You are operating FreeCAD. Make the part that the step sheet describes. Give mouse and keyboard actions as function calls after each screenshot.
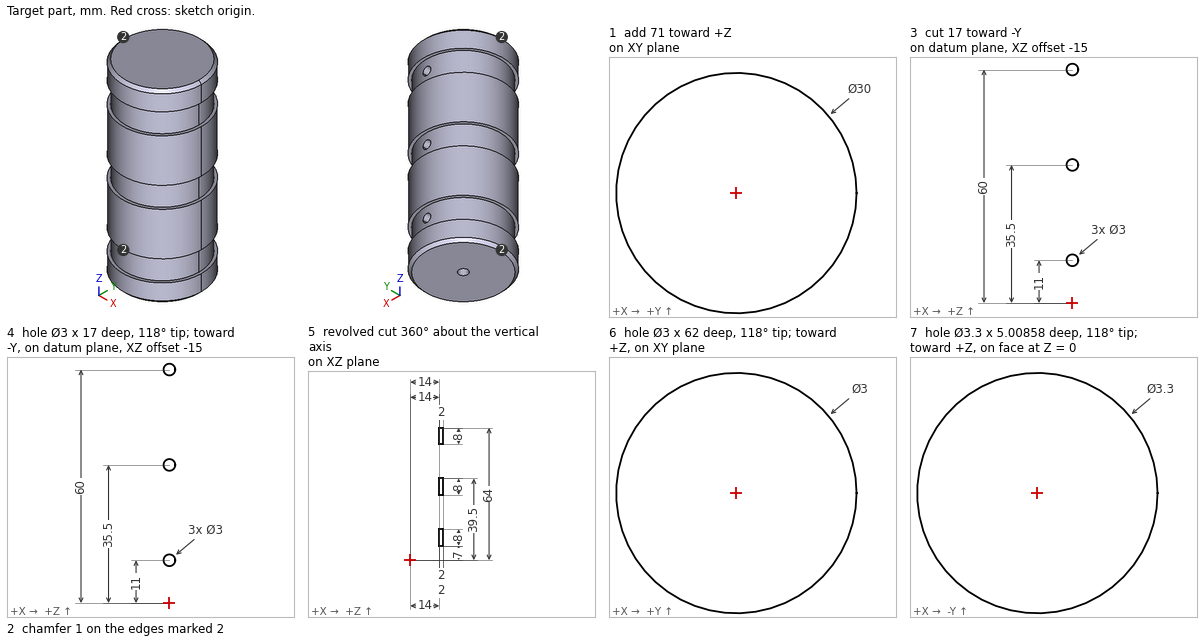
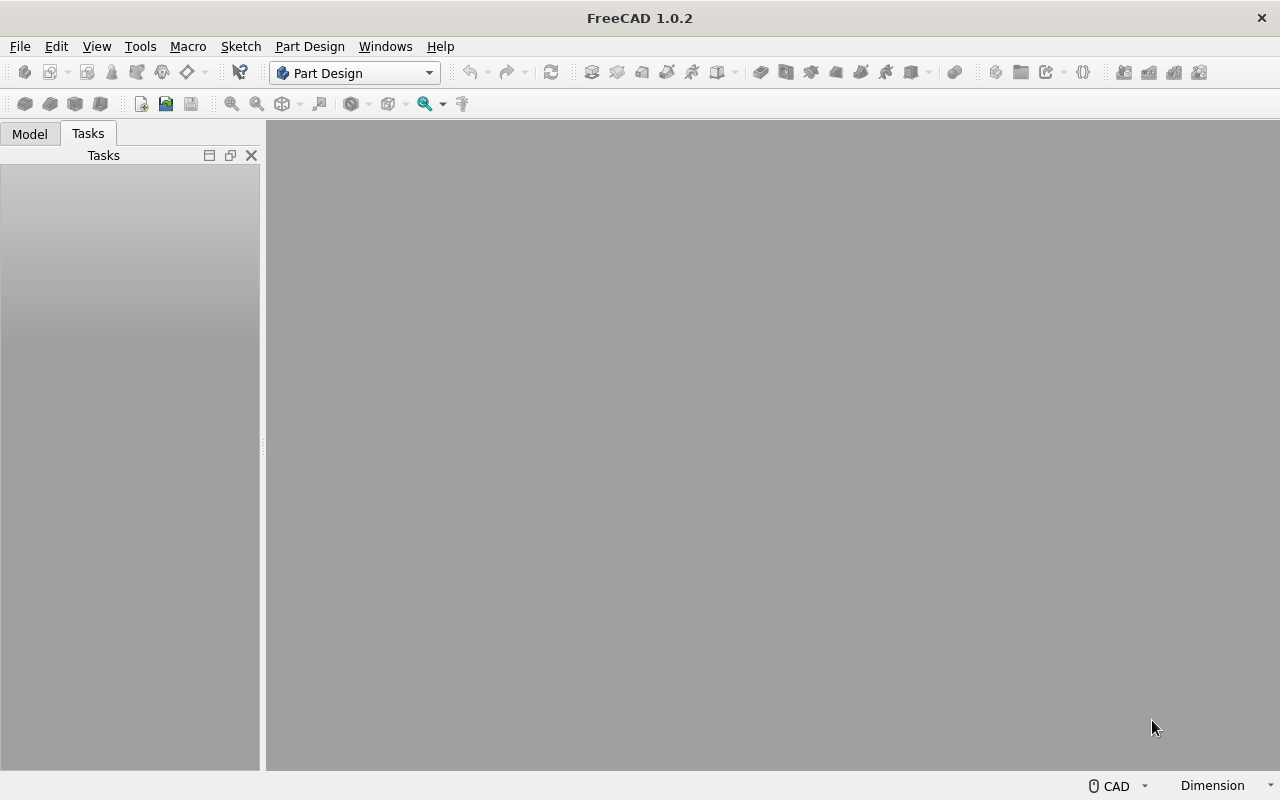
click(141, 104)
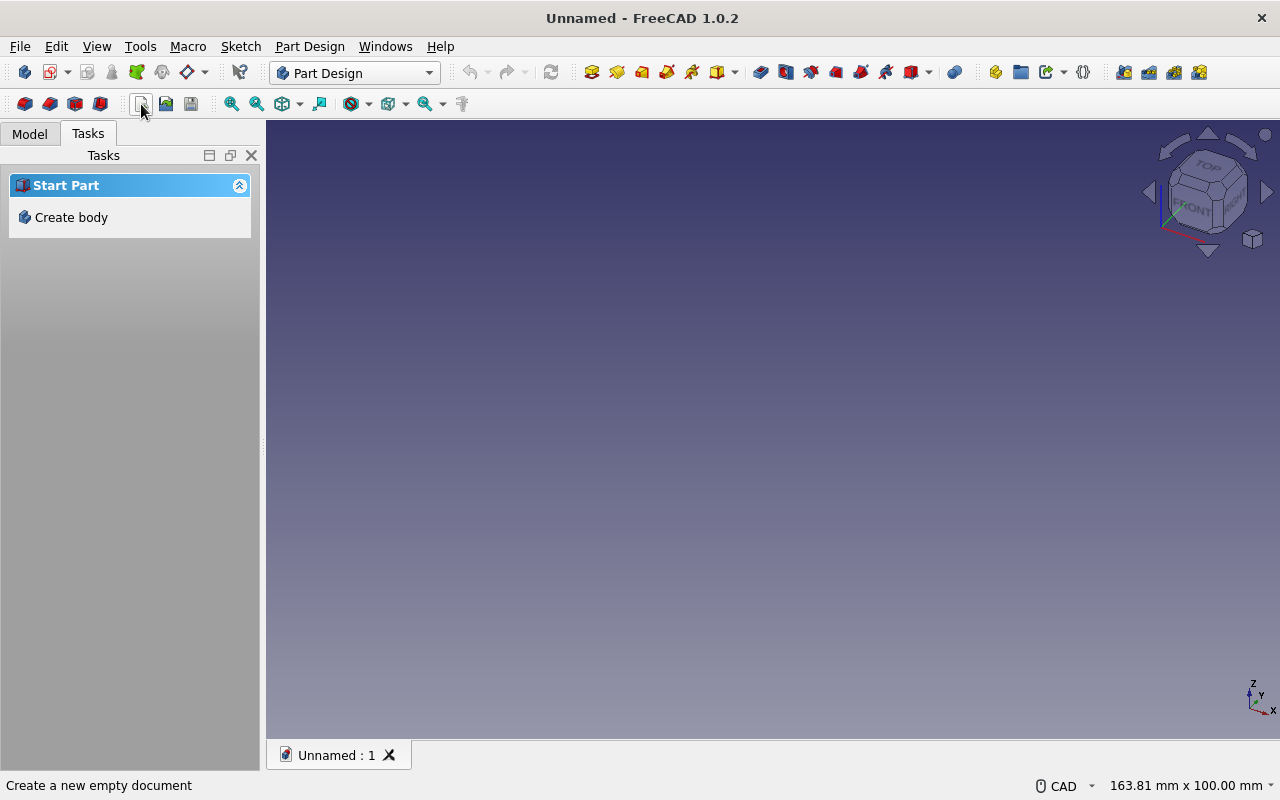
click(50, 72)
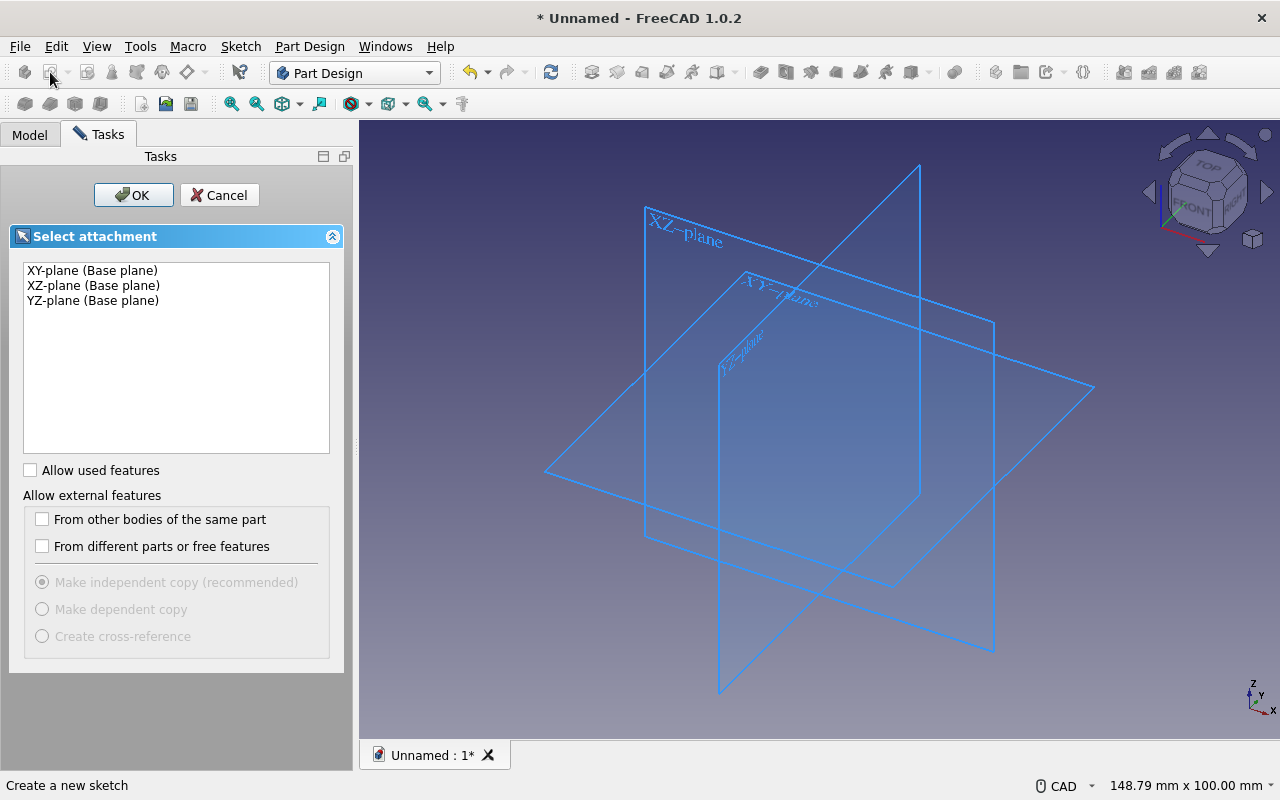
click(84, 270)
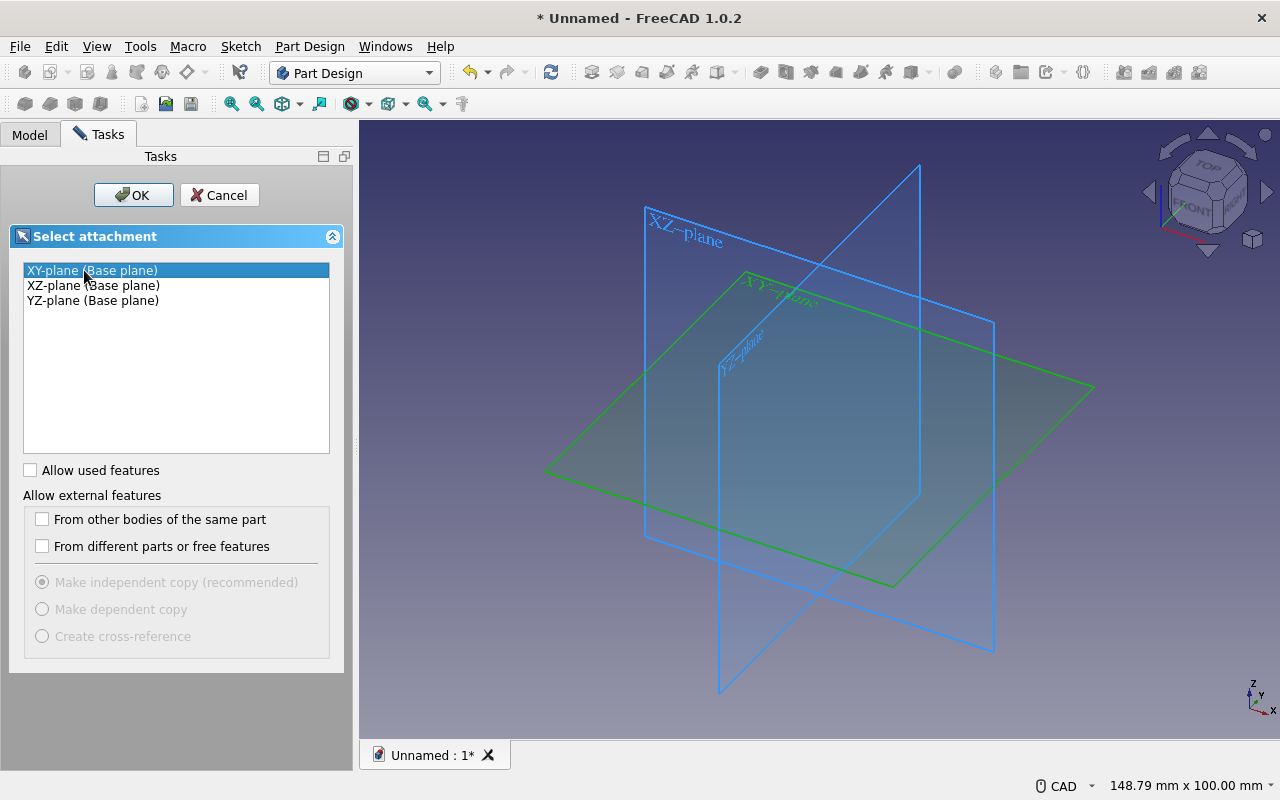
click(134, 195)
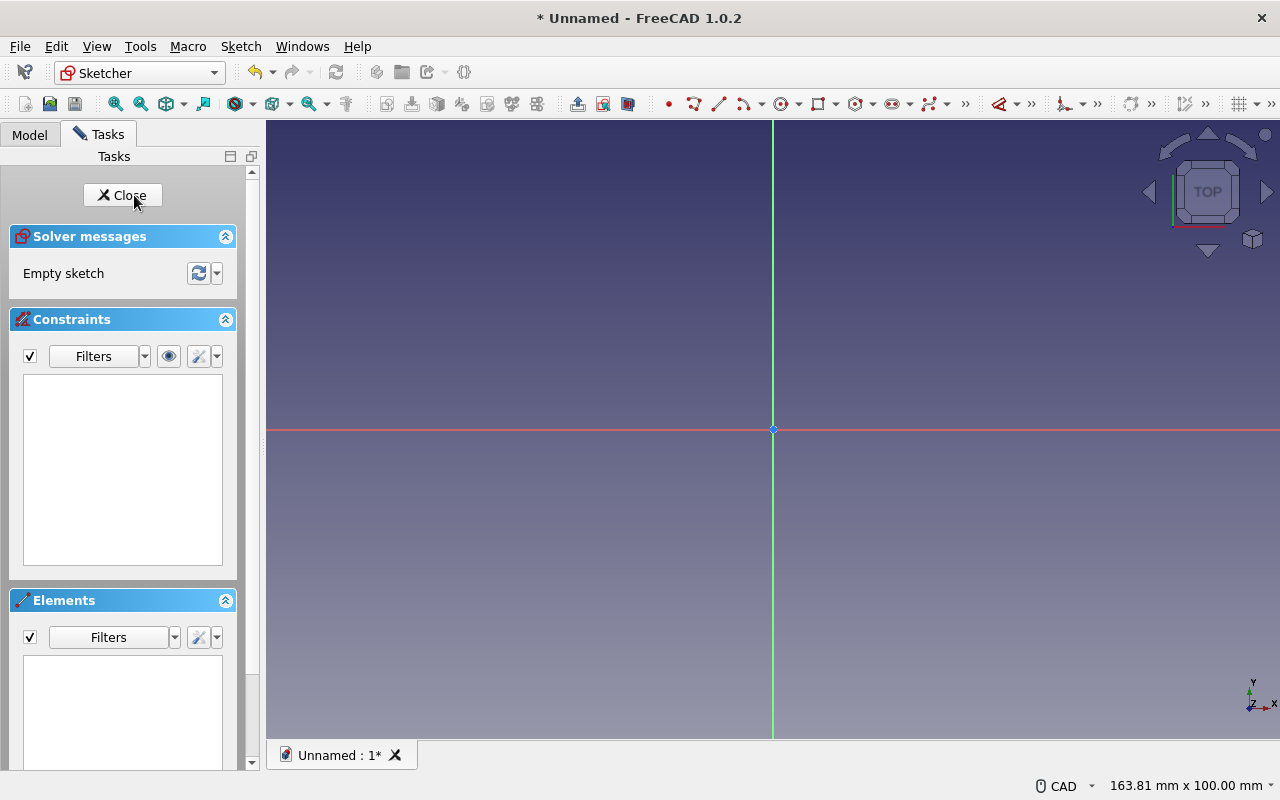
scroll(829, 430, up, 4)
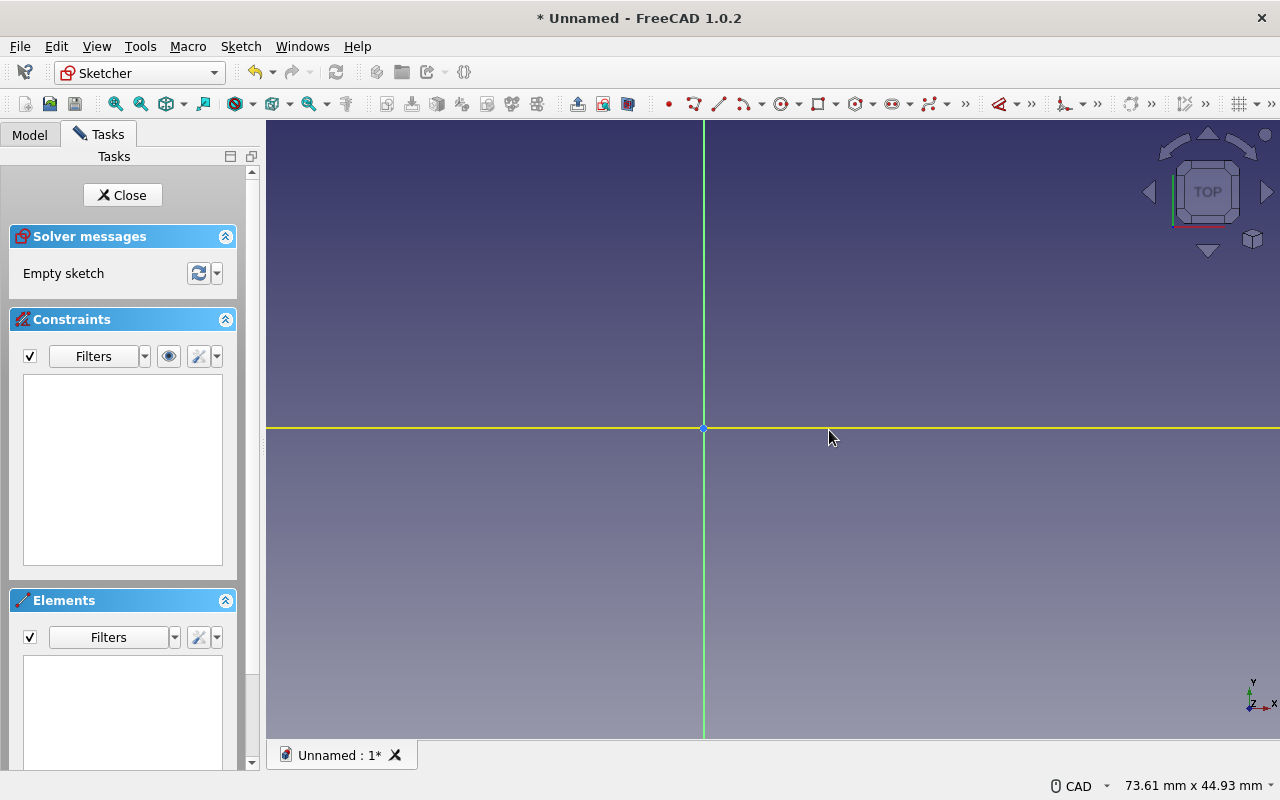
click(780, 104)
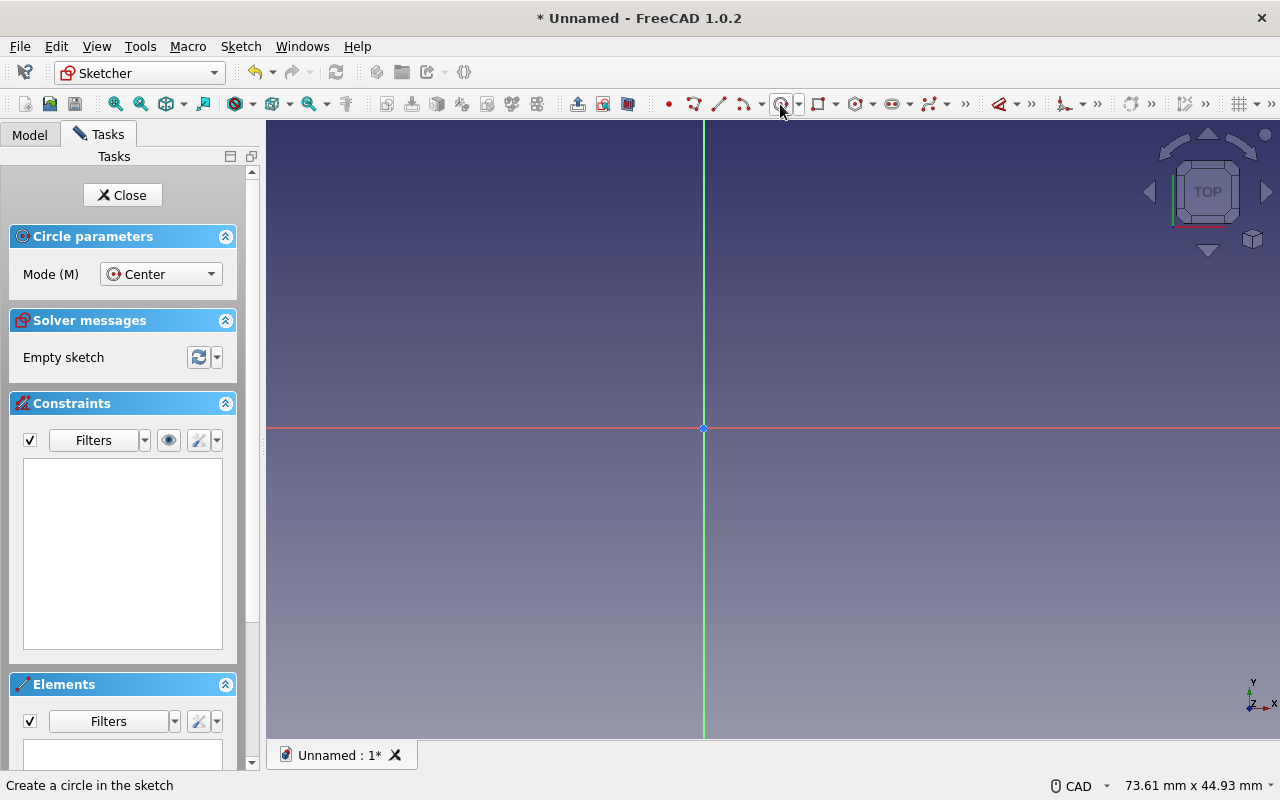
click(704, 428)
move(850, 282)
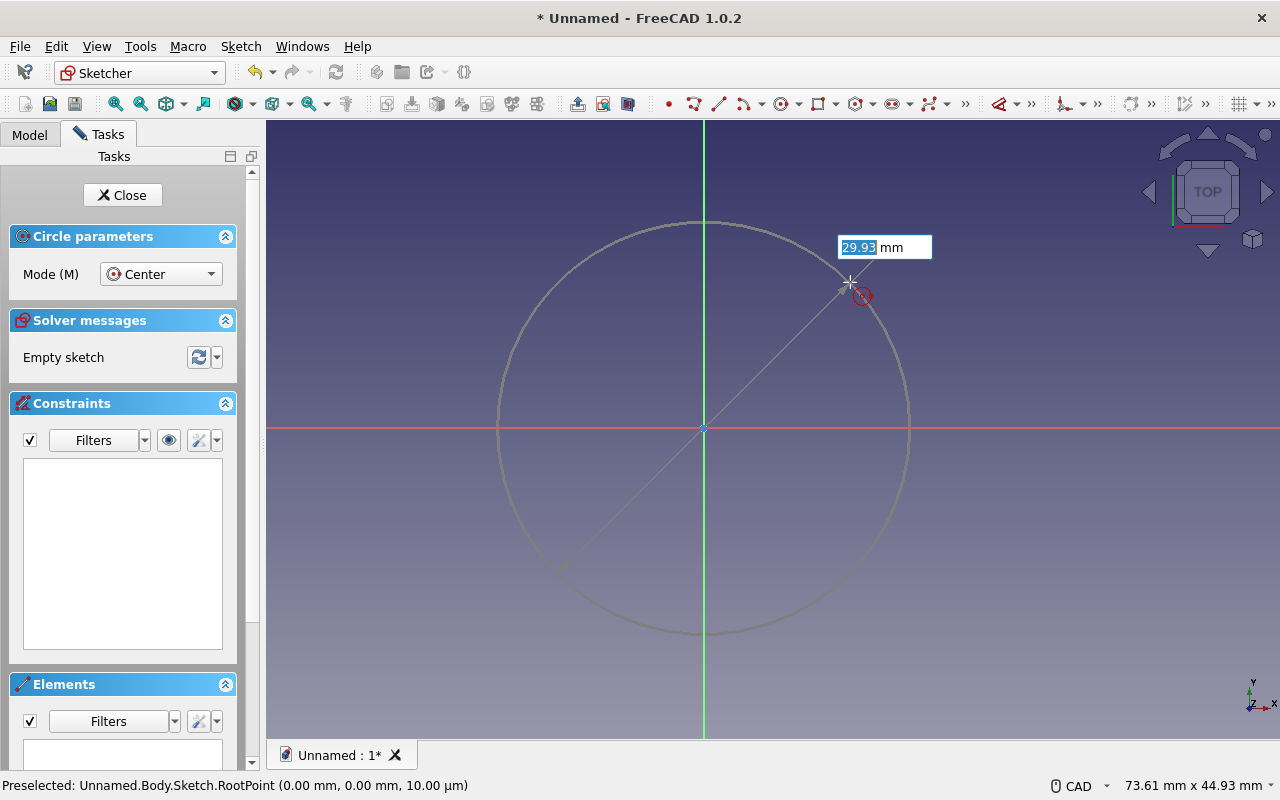
text(30)
key(Return)
key(Escape)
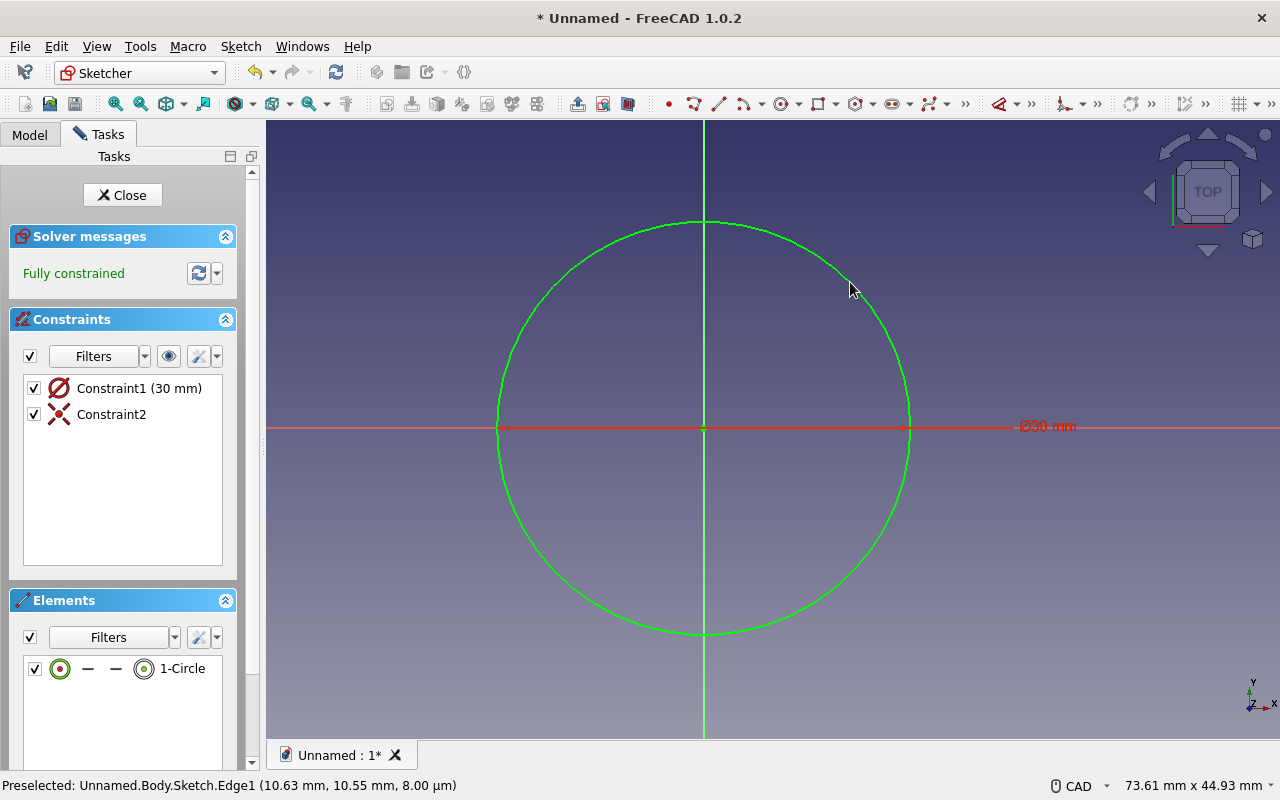
click(123, 195)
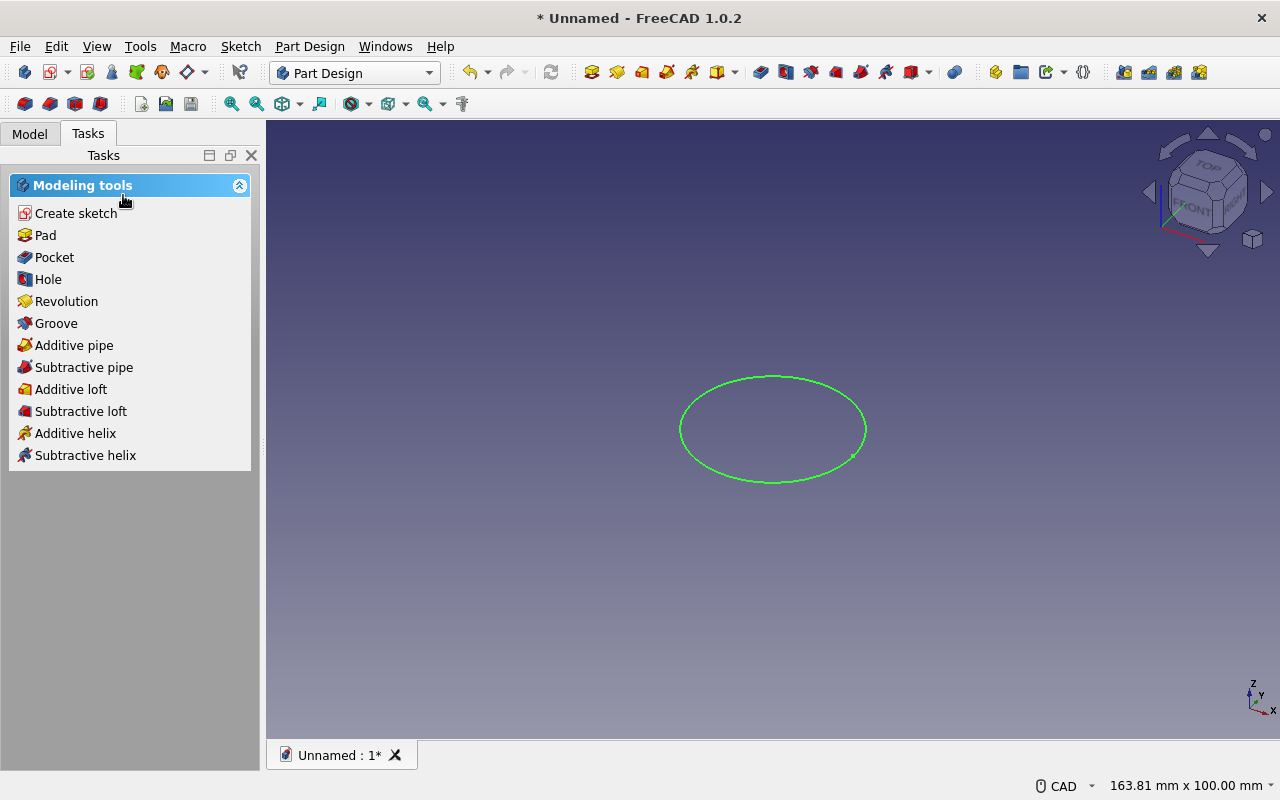
click(592, 72)